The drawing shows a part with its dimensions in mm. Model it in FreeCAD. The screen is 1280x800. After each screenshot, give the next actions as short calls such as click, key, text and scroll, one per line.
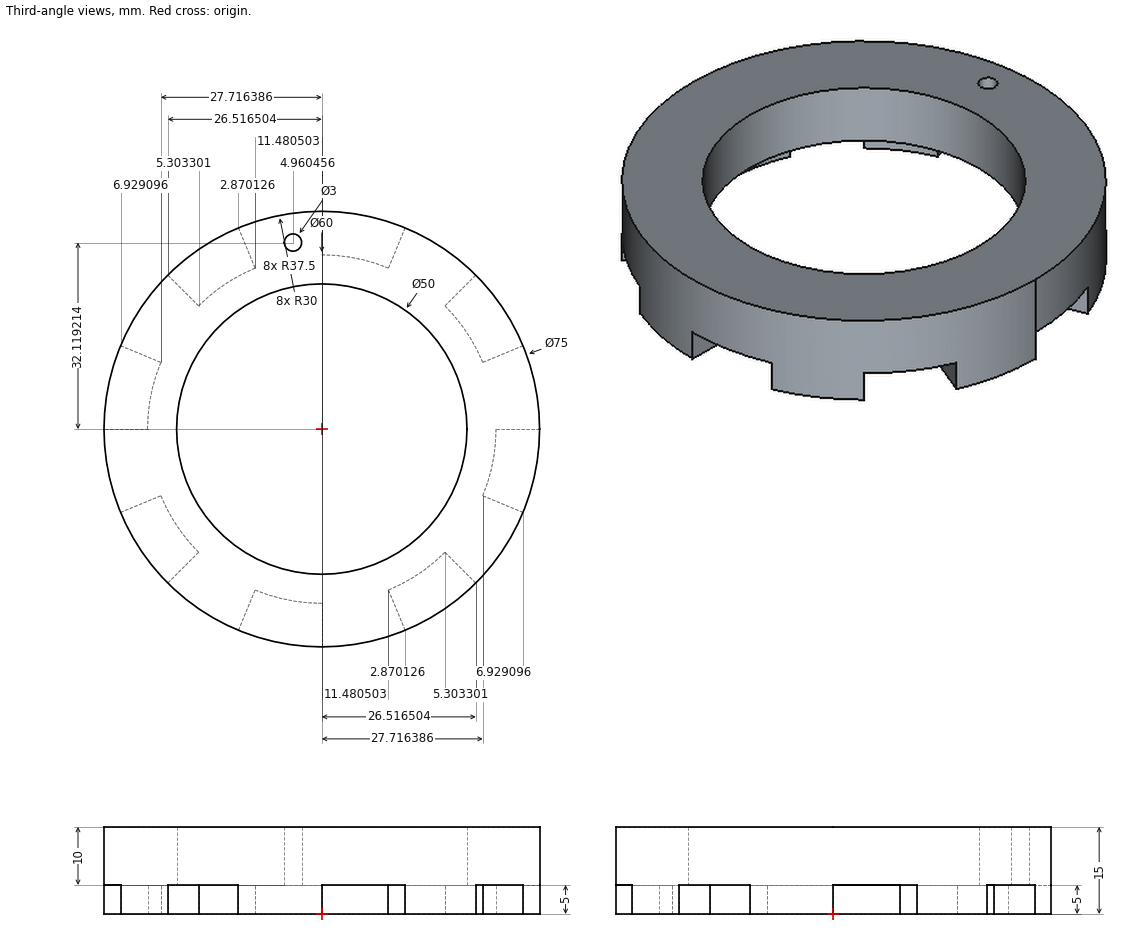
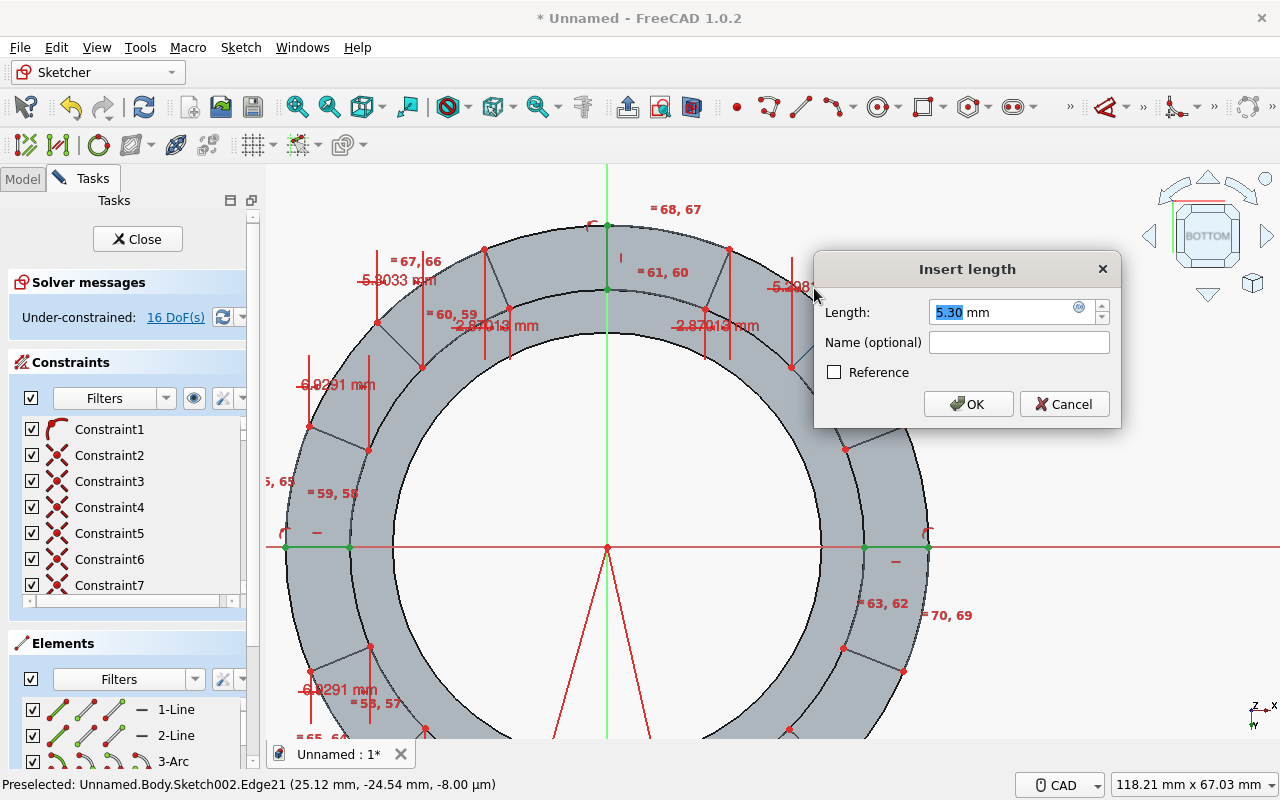
text(5.303301)
key(Return)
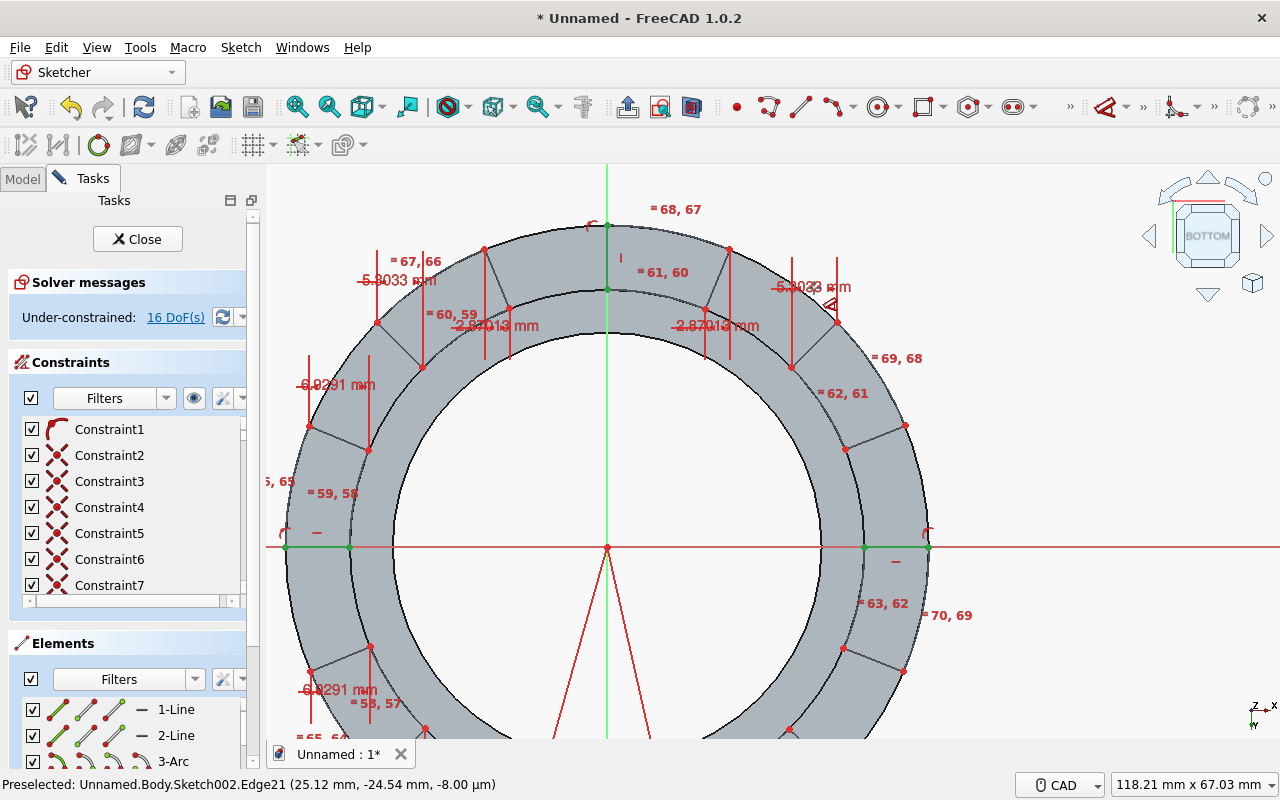
click(863, 443)
click(862, 392)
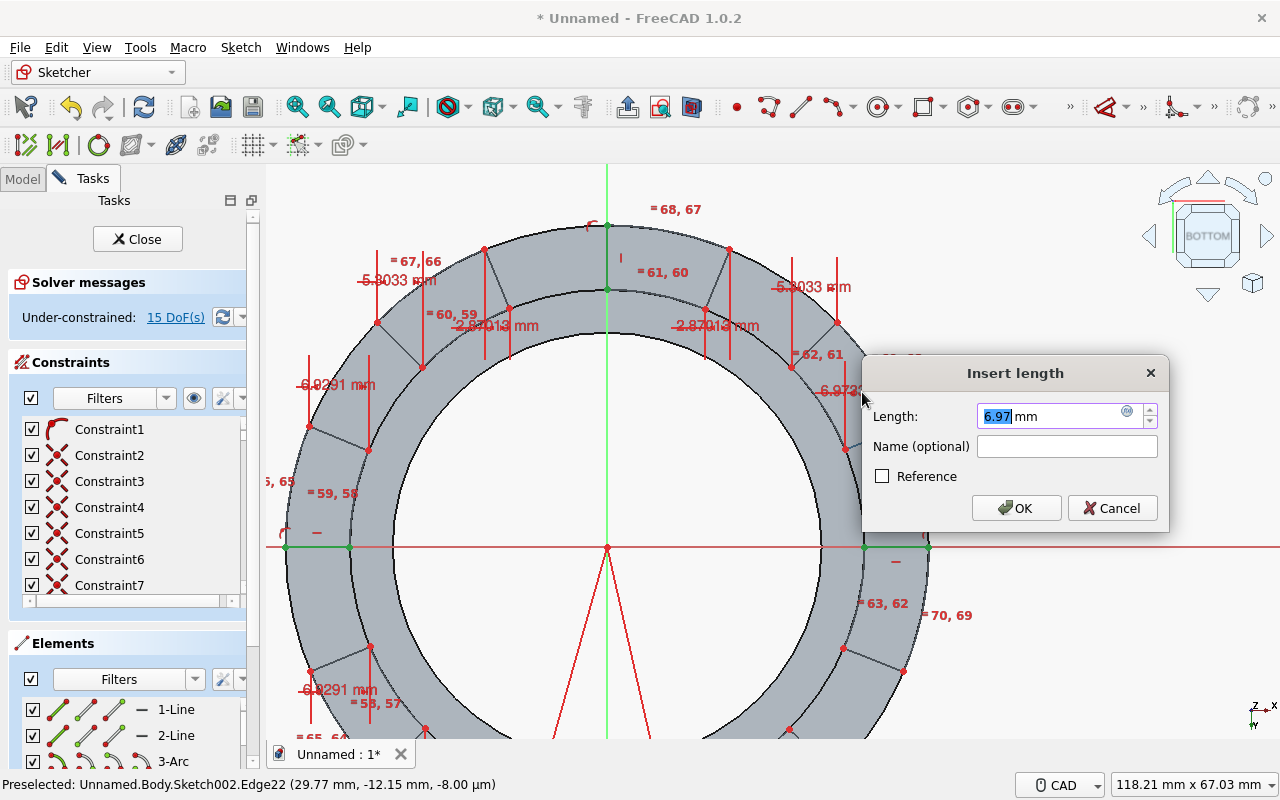
text(6.929096)
key(Return)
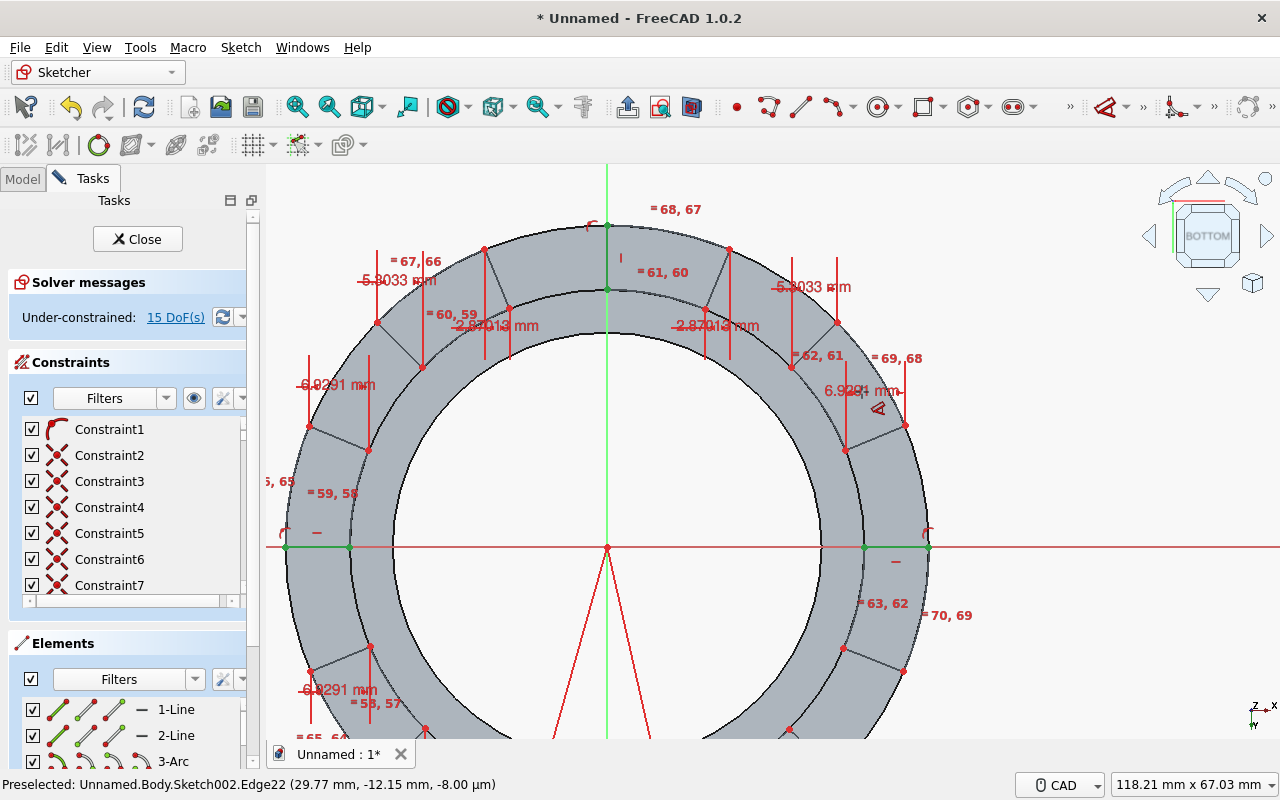
click(862, 655)
click(874, 706)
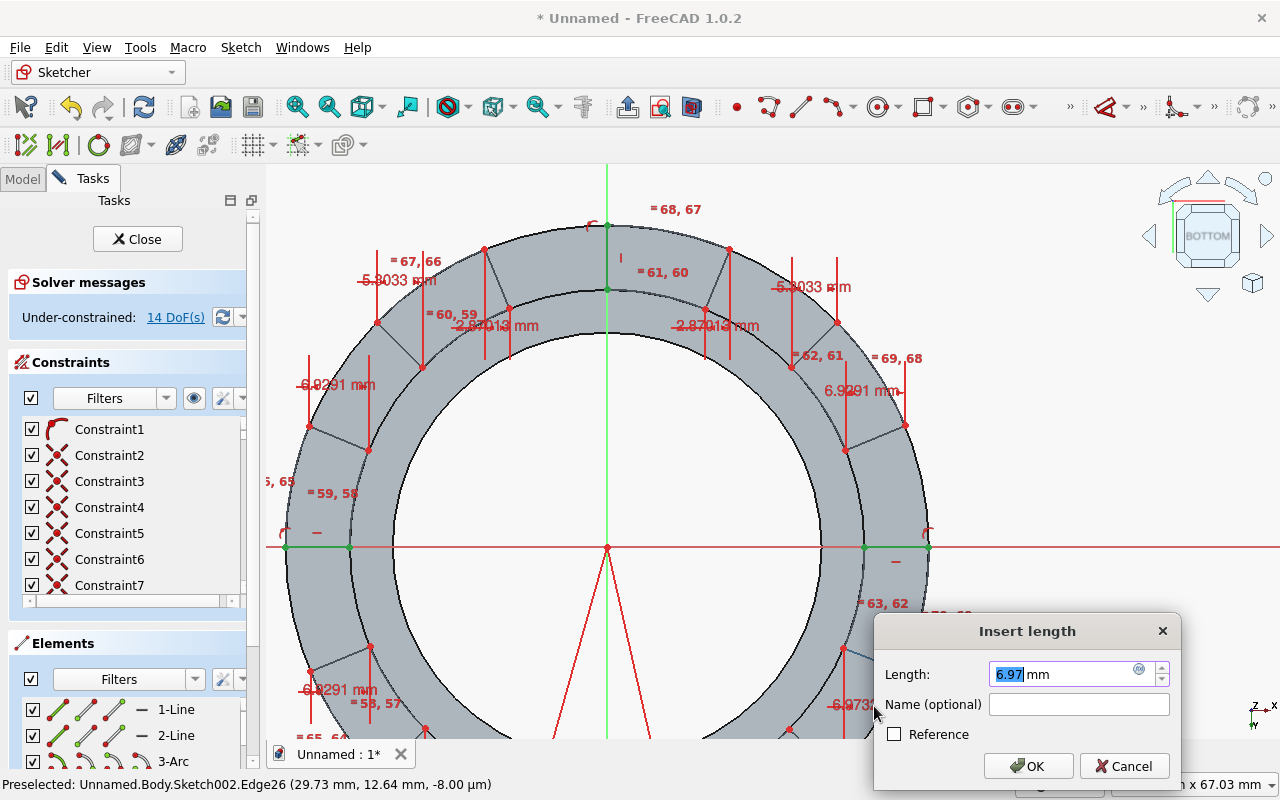
text(6.929096)
key(Return)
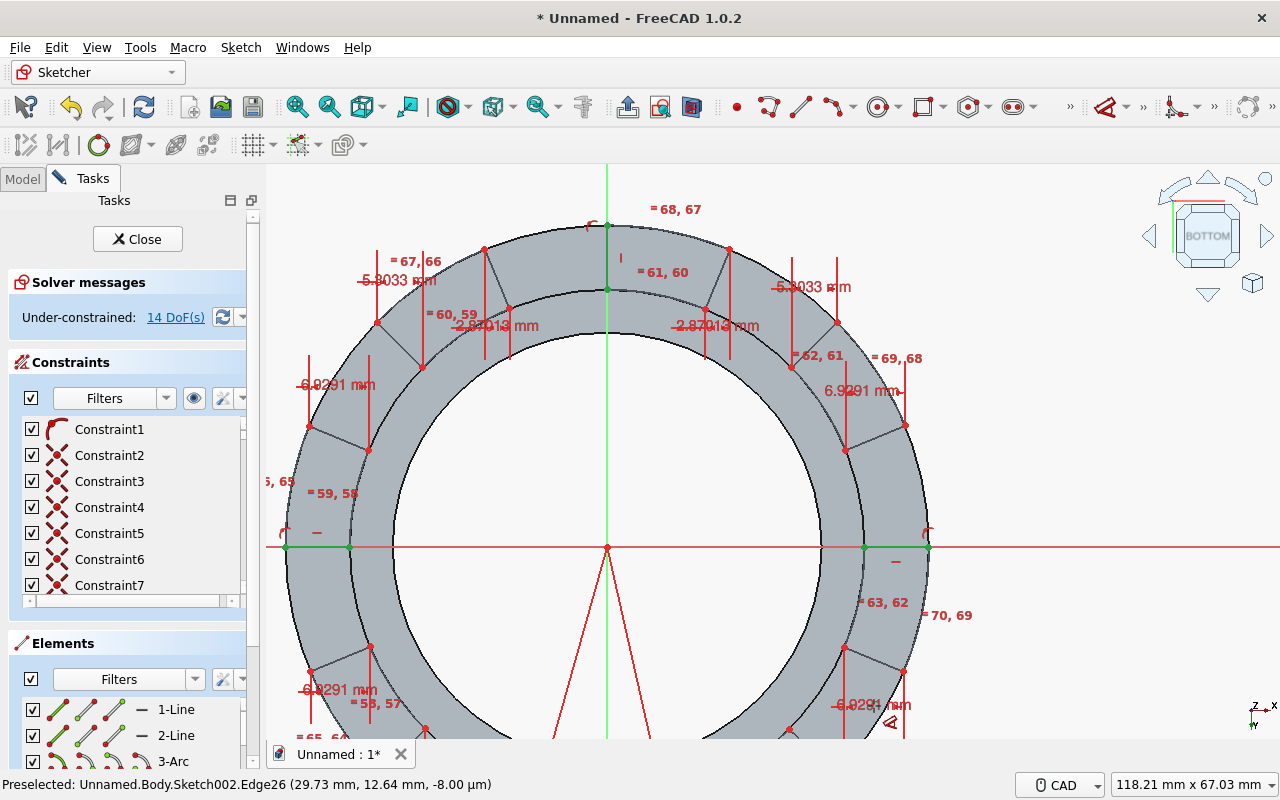
scroll(823, 335, down, 3)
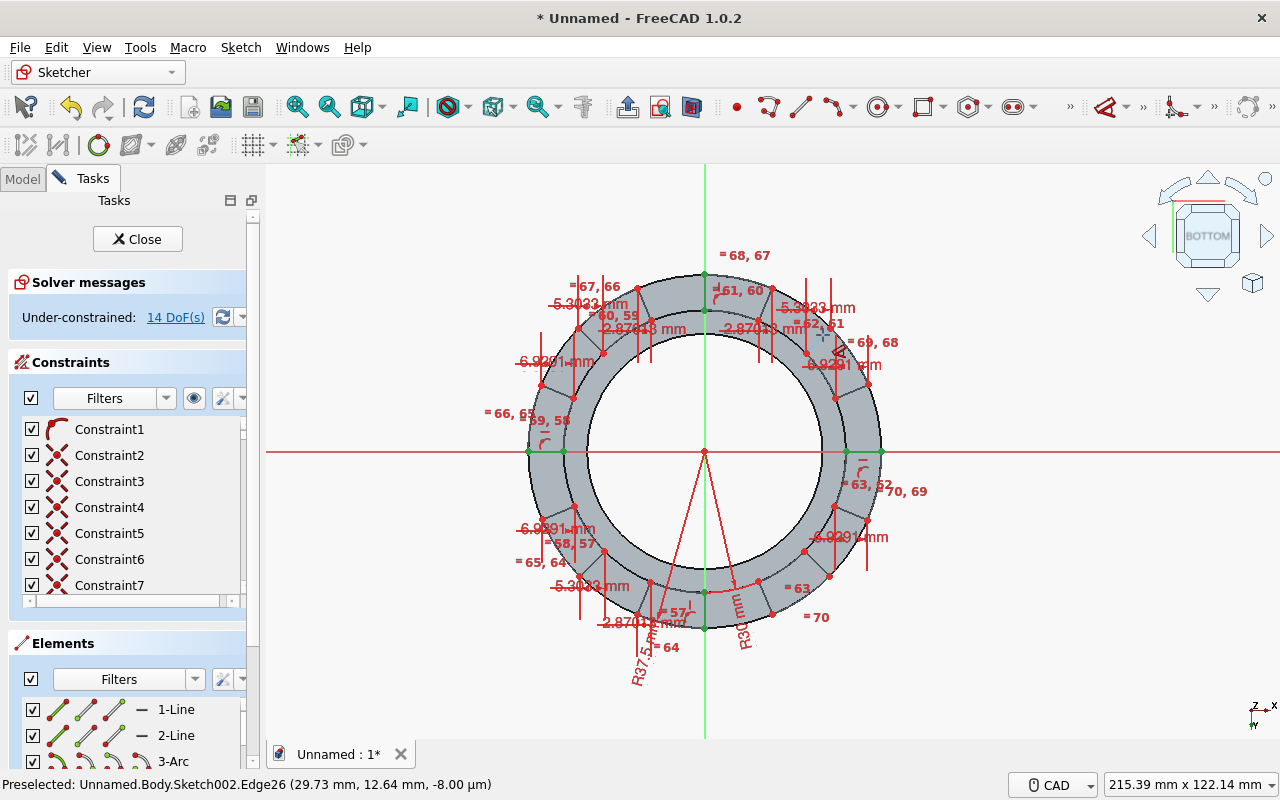
scroll(822, 569, up, 3)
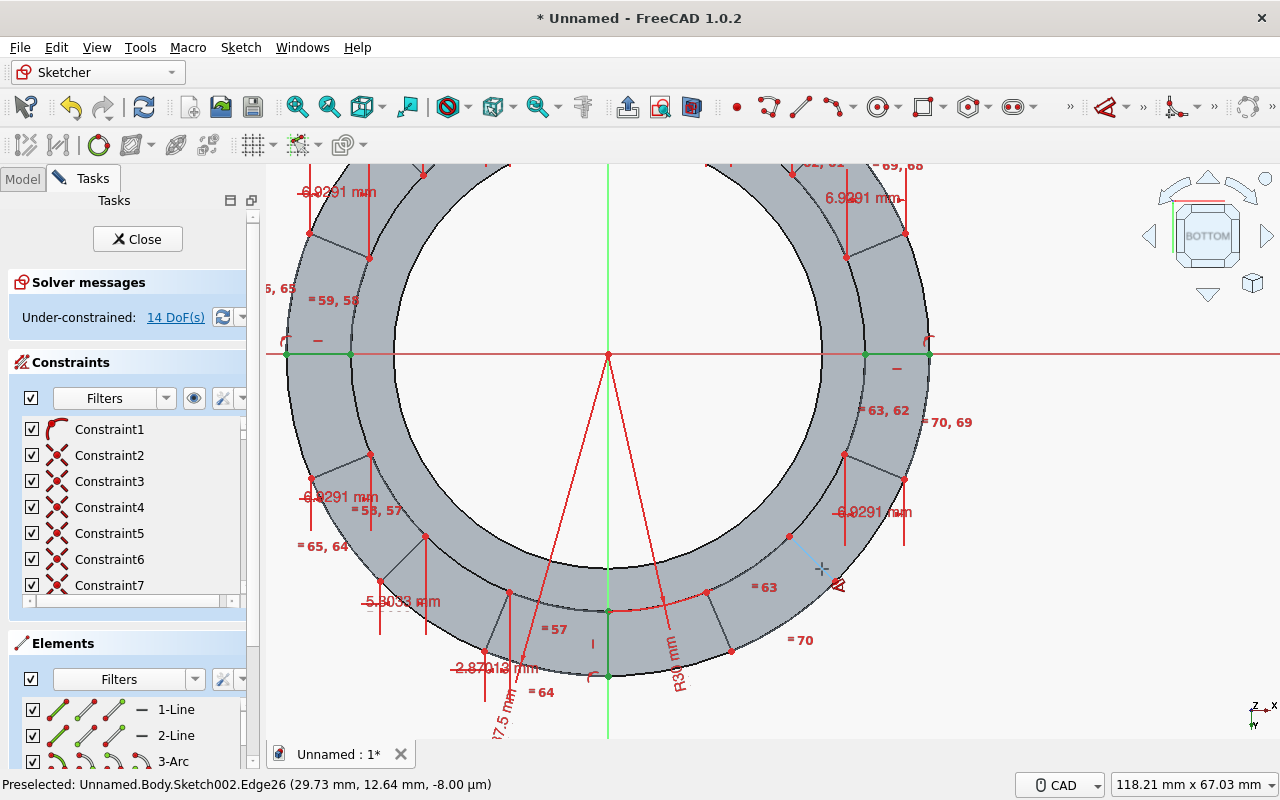
click(822, 568)
click(823, 616)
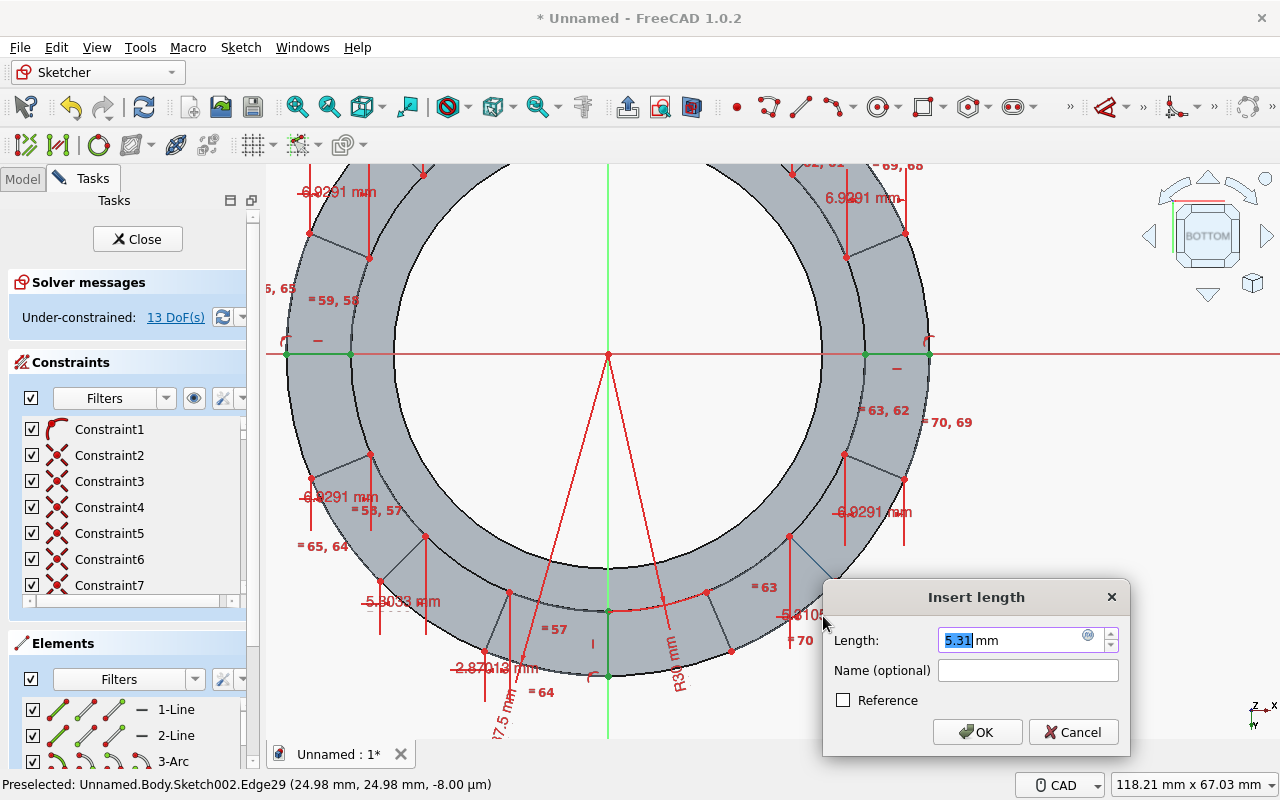
text(5.303301)
key(Return)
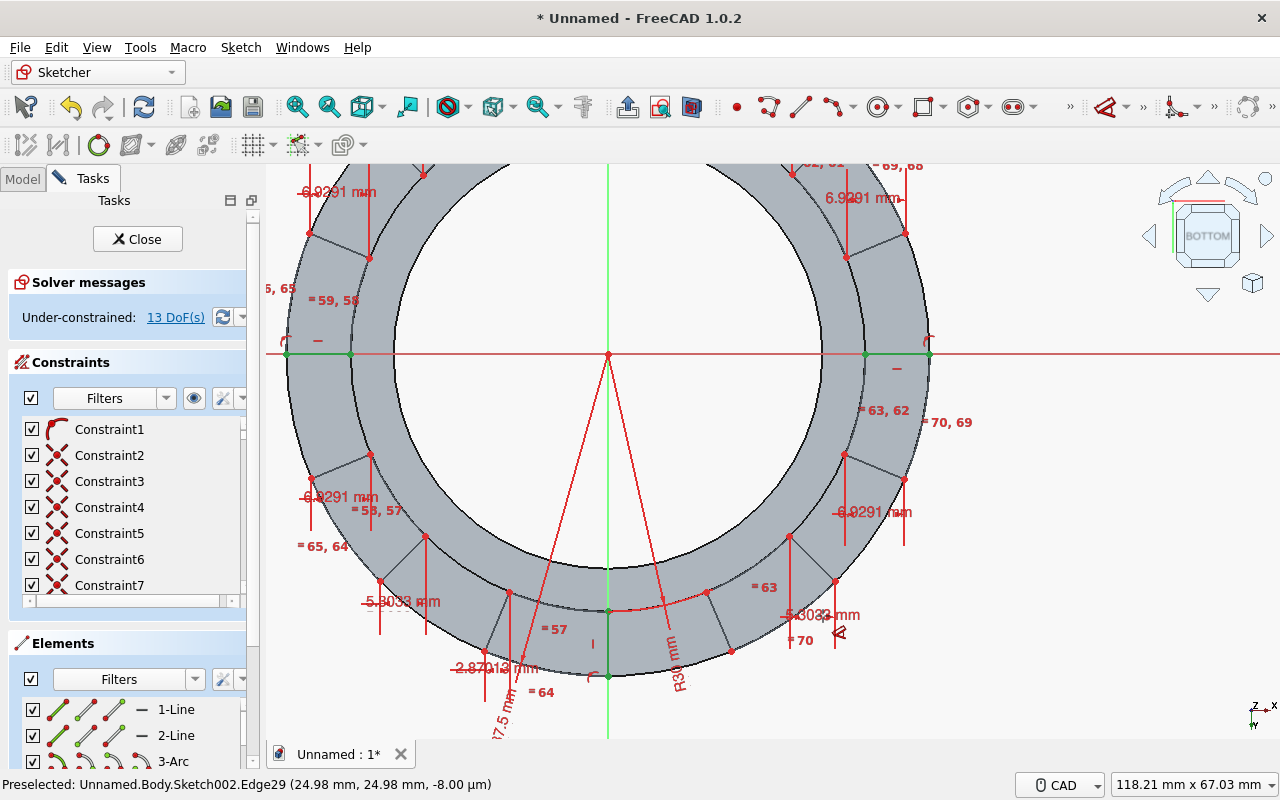
scroll(714, 610, up, 3)